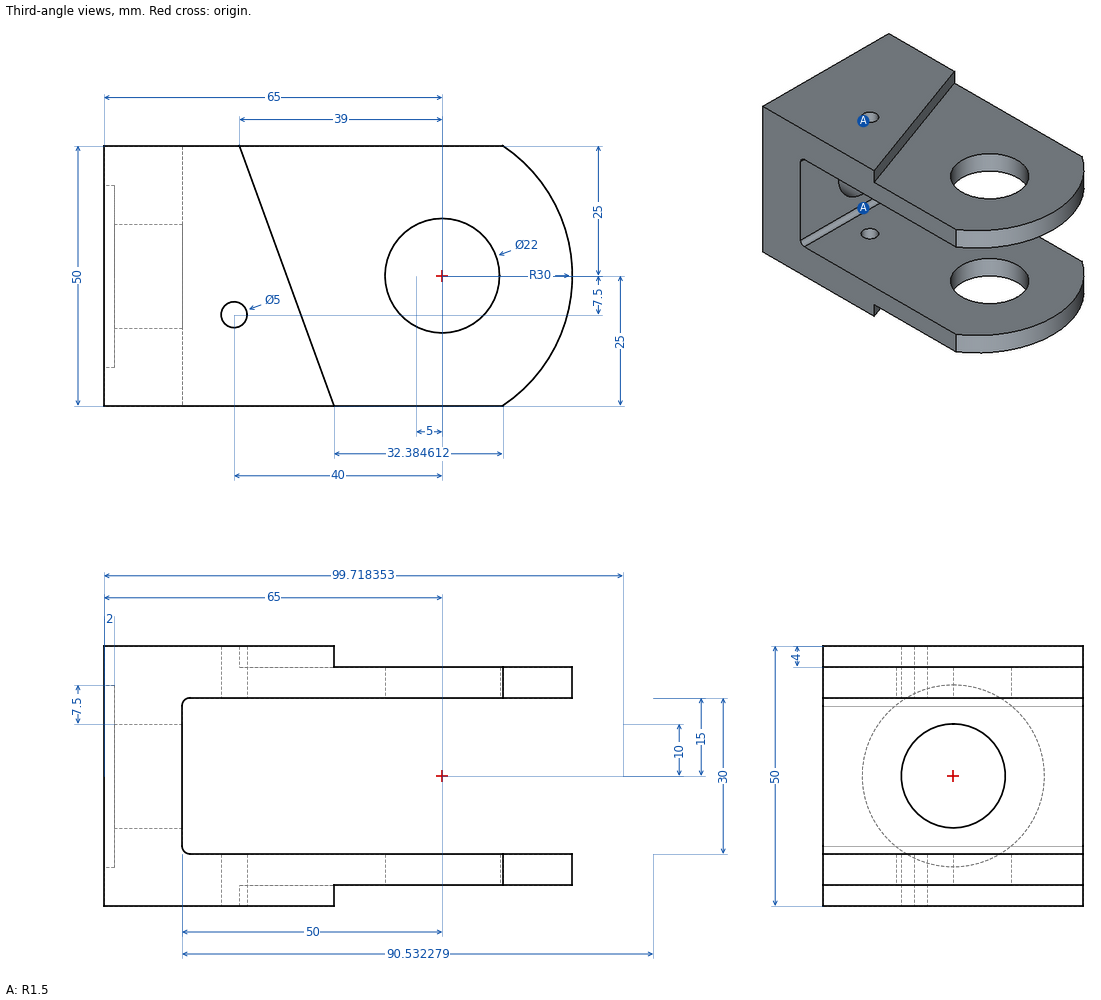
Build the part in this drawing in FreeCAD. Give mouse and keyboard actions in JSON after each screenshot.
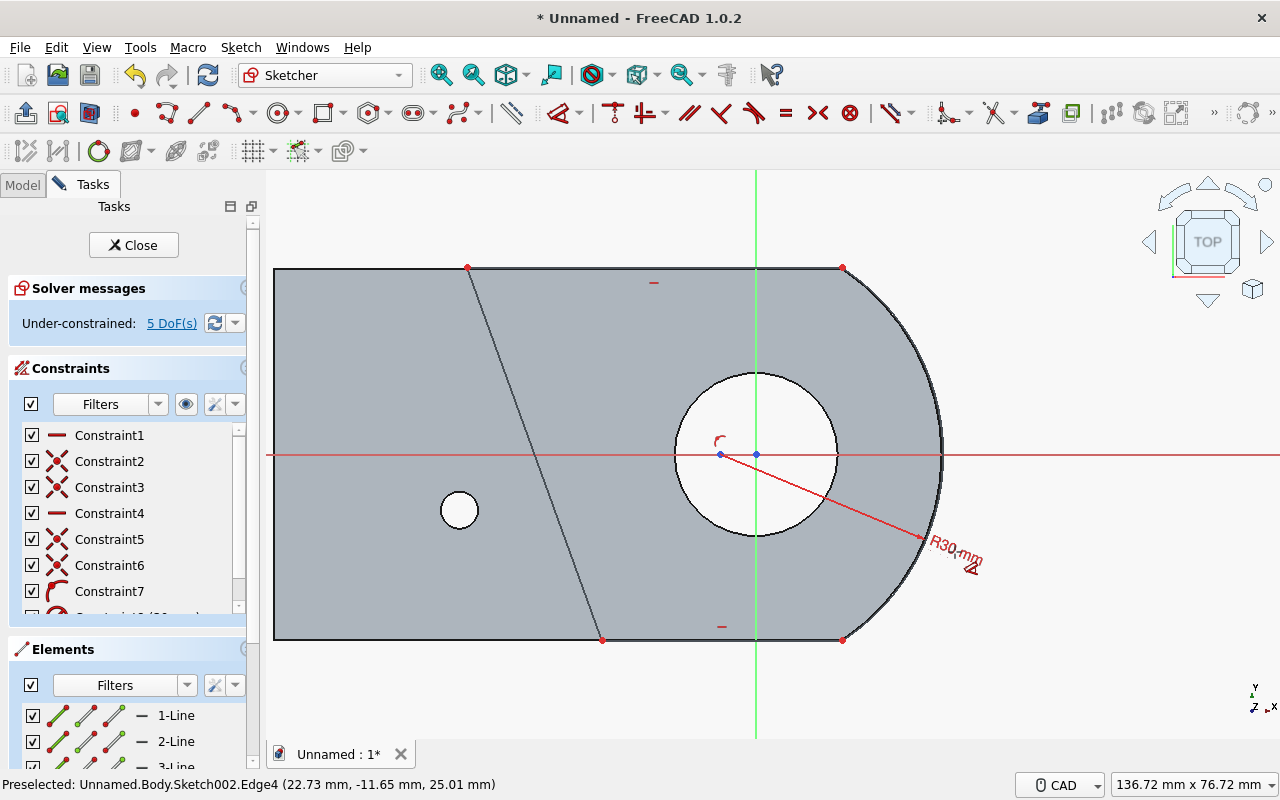
{"action": "left_click", "coordinate": [721, 454]}
{"action": "left_click", "coordinate": [738, 488]}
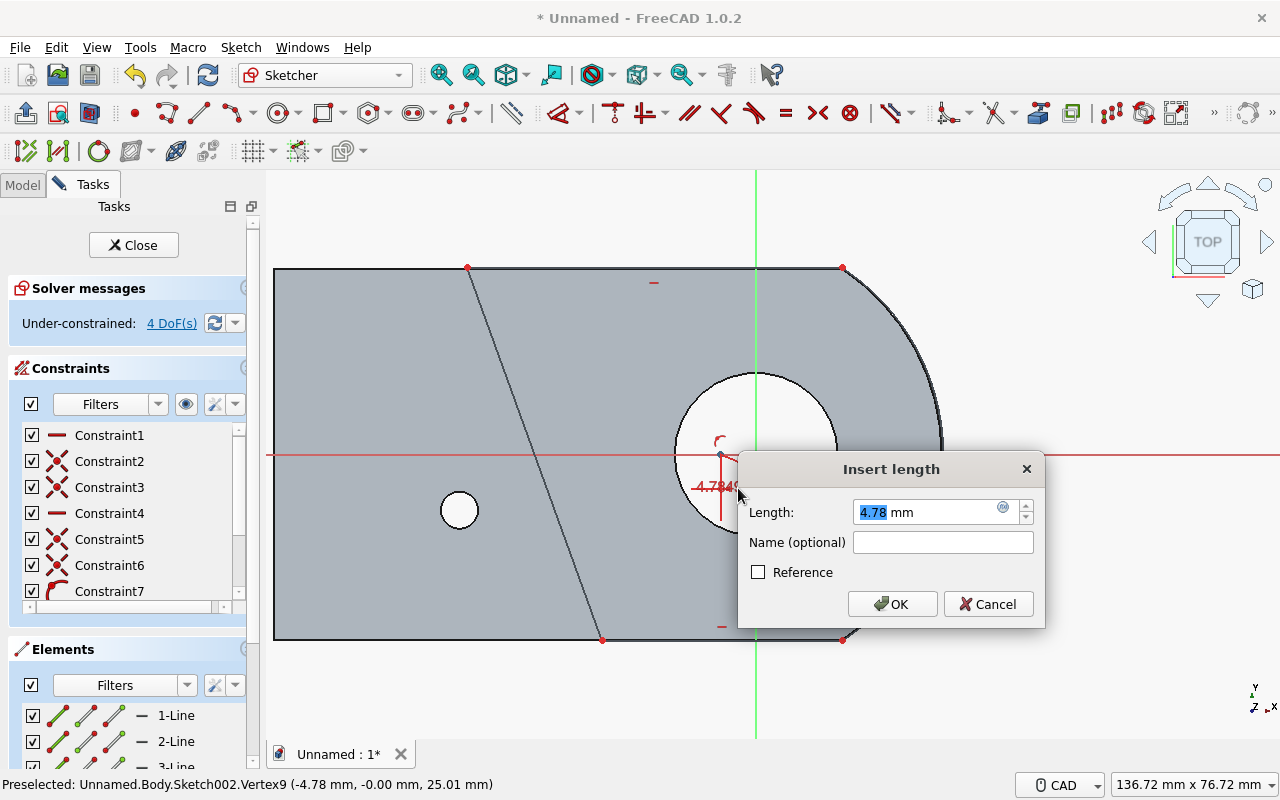
{"action": "type", "text": "5"}
{"action": "key", "text": "Return"}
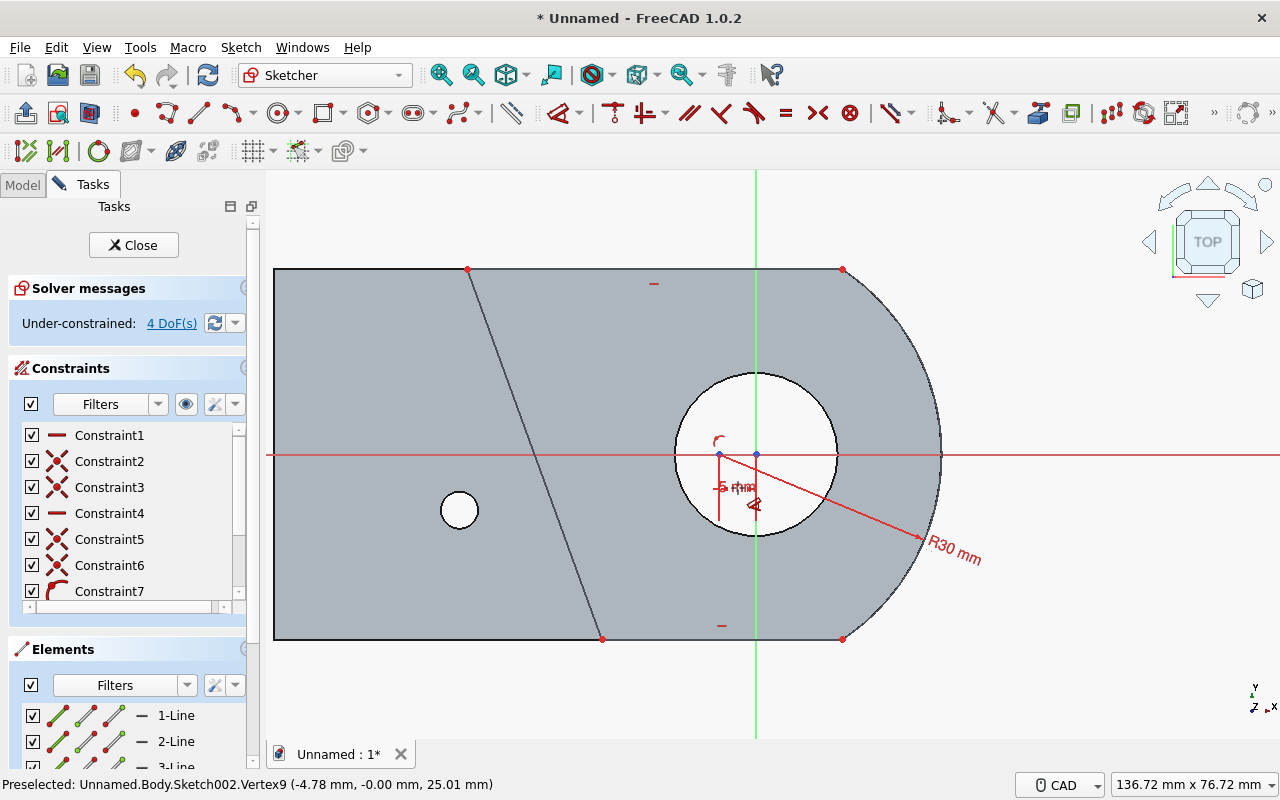
{"action": "left_click", "coordinate": [842, 269]}
{"action": "left_click", "coordinate": [876, 362]}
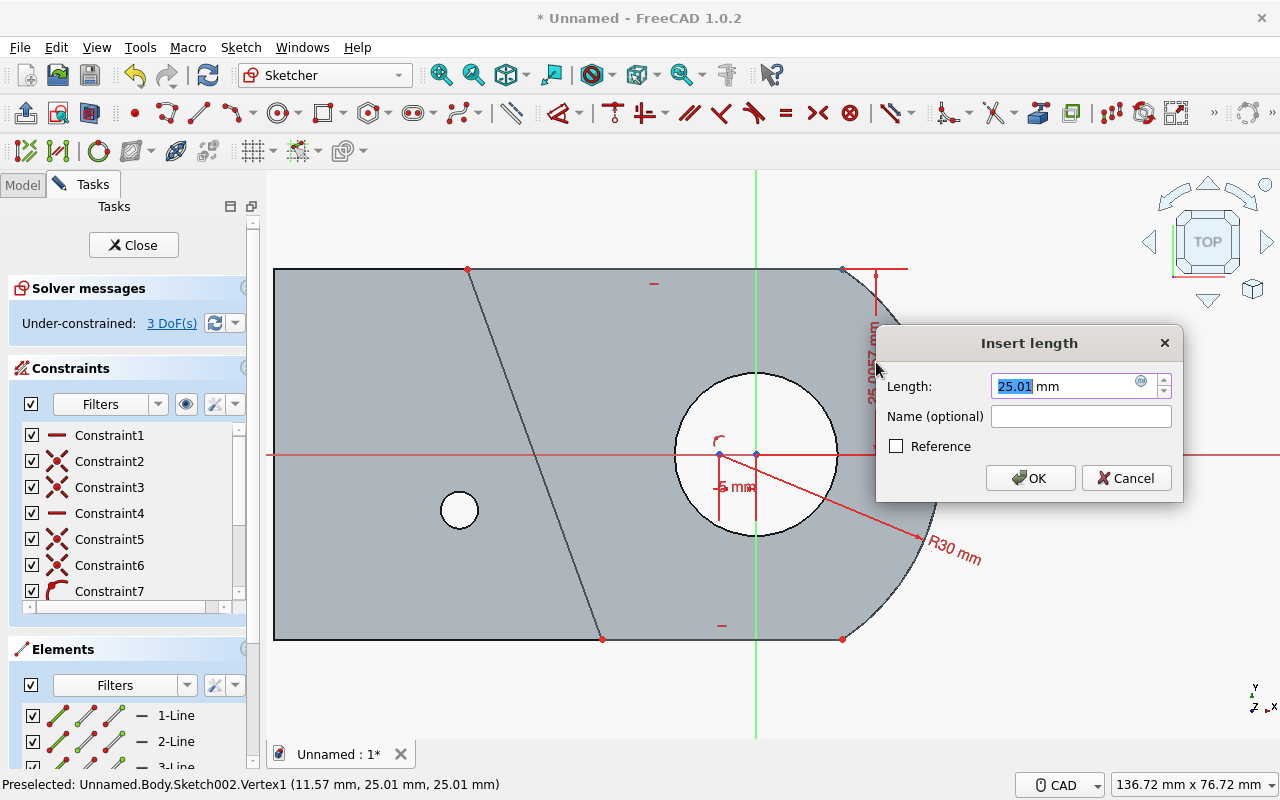
{"action": "type", "text": "25"}
{"action": "key", "text": "Return"}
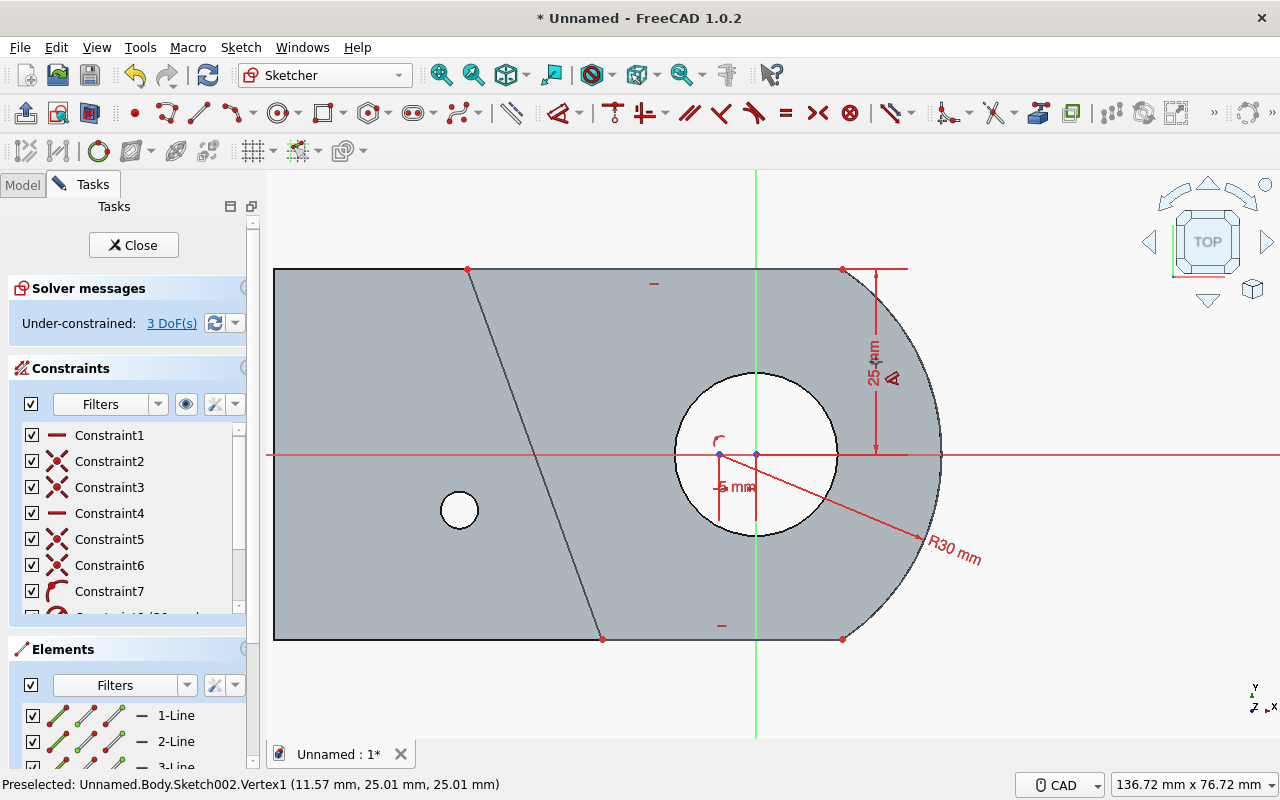
{"action": "left_click", "coordinate": [467, 269]}
{"action": "left_click", "coordinate": [612, 235]}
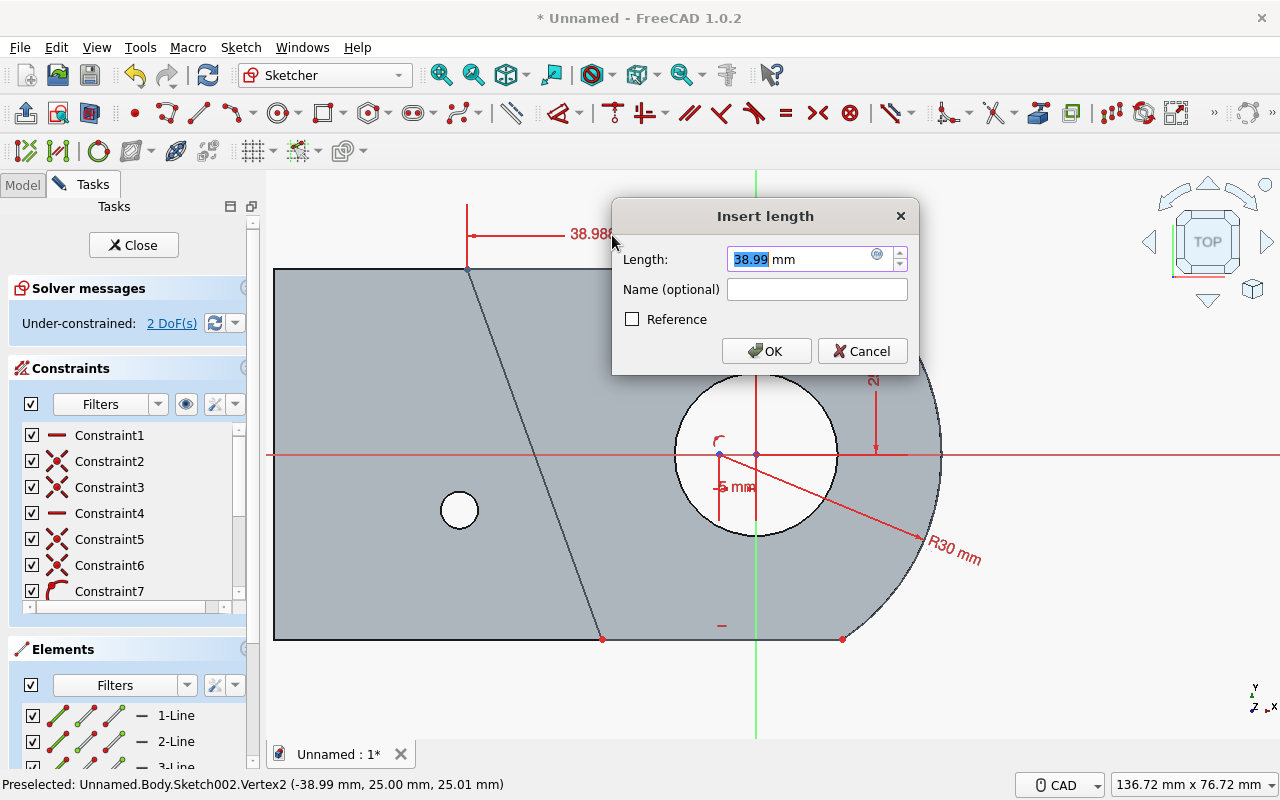
{"action": "type", "text": "39"}
{"action": "key", "text": "Return"}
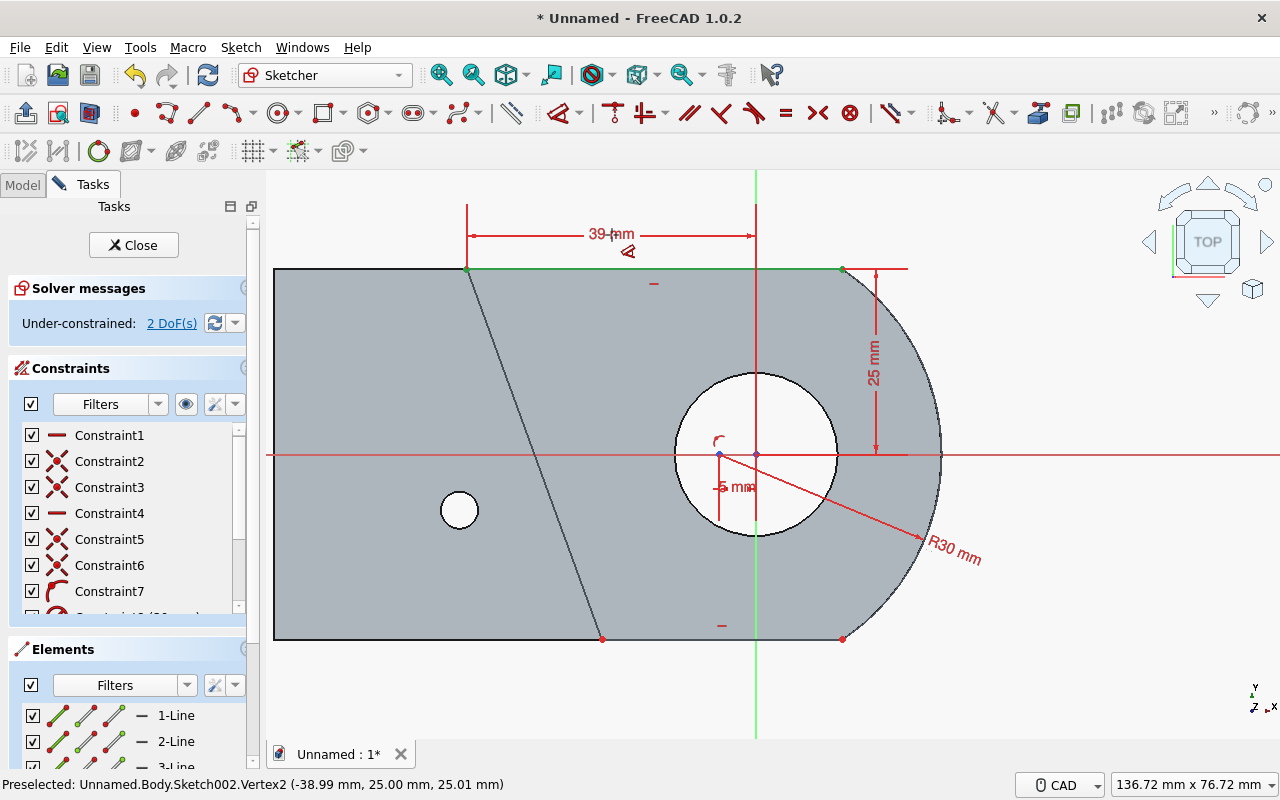
{"action": "left_click", "coordinate": [602, 640]}
{"action": "left_click", "coordinate": [568, 505]}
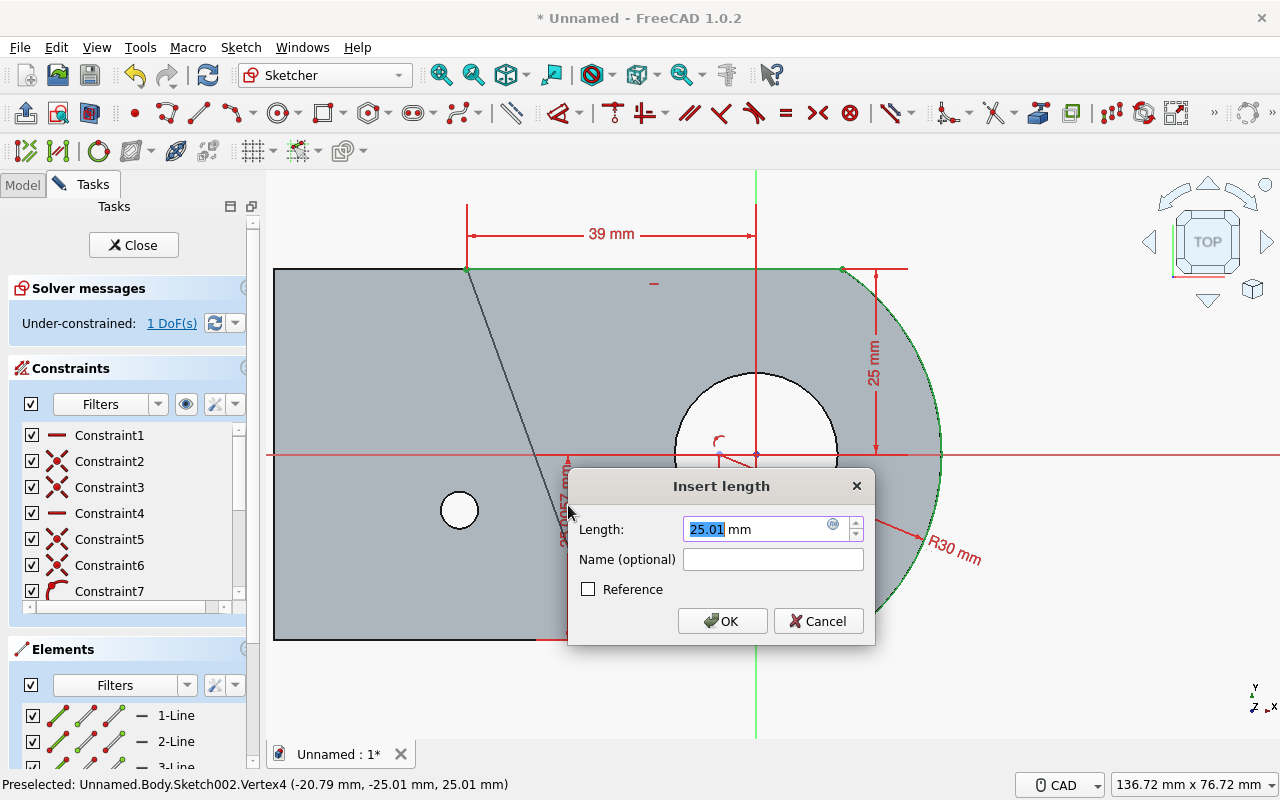
{"action": "type", "text": "25"}
{"action": "key", "text": "Return"}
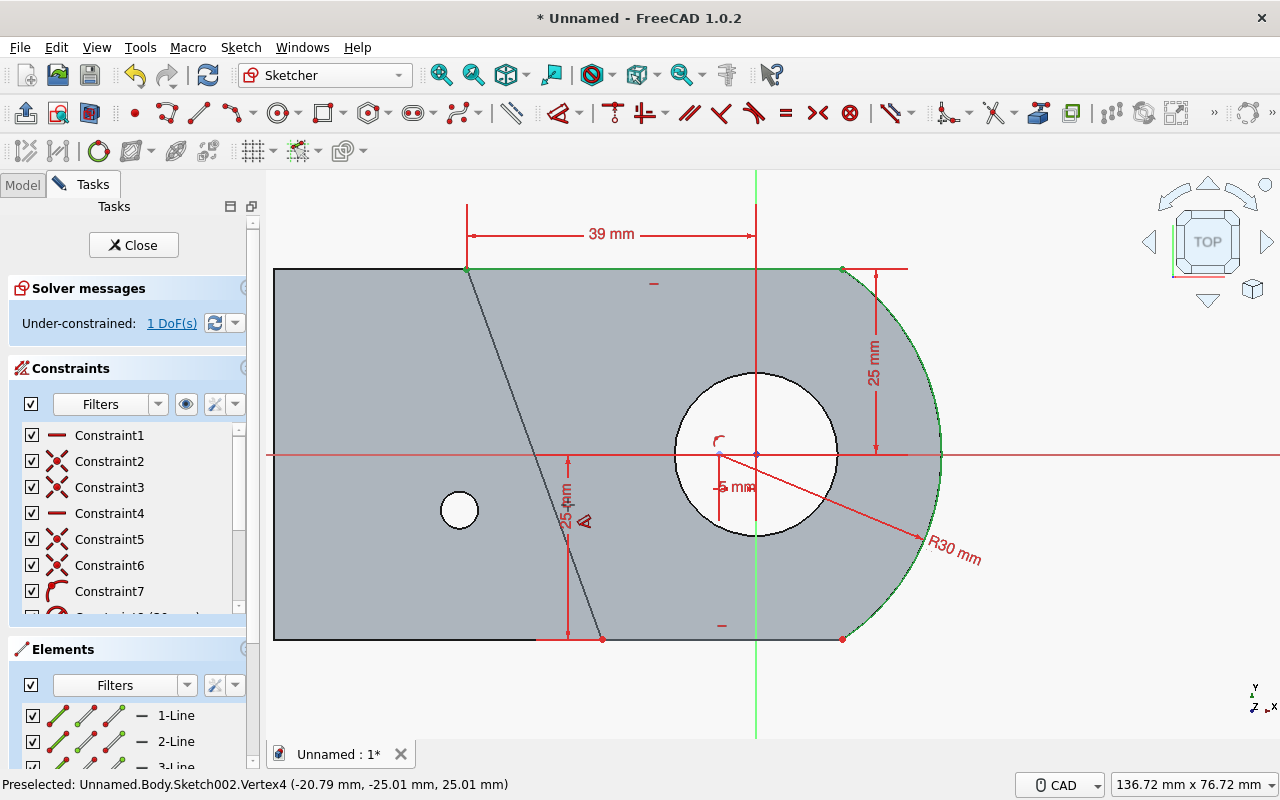
{"action": "left_click", "coordinate": [674, 640]}
{"action": "left_click", "coordinate": [722, 674]}